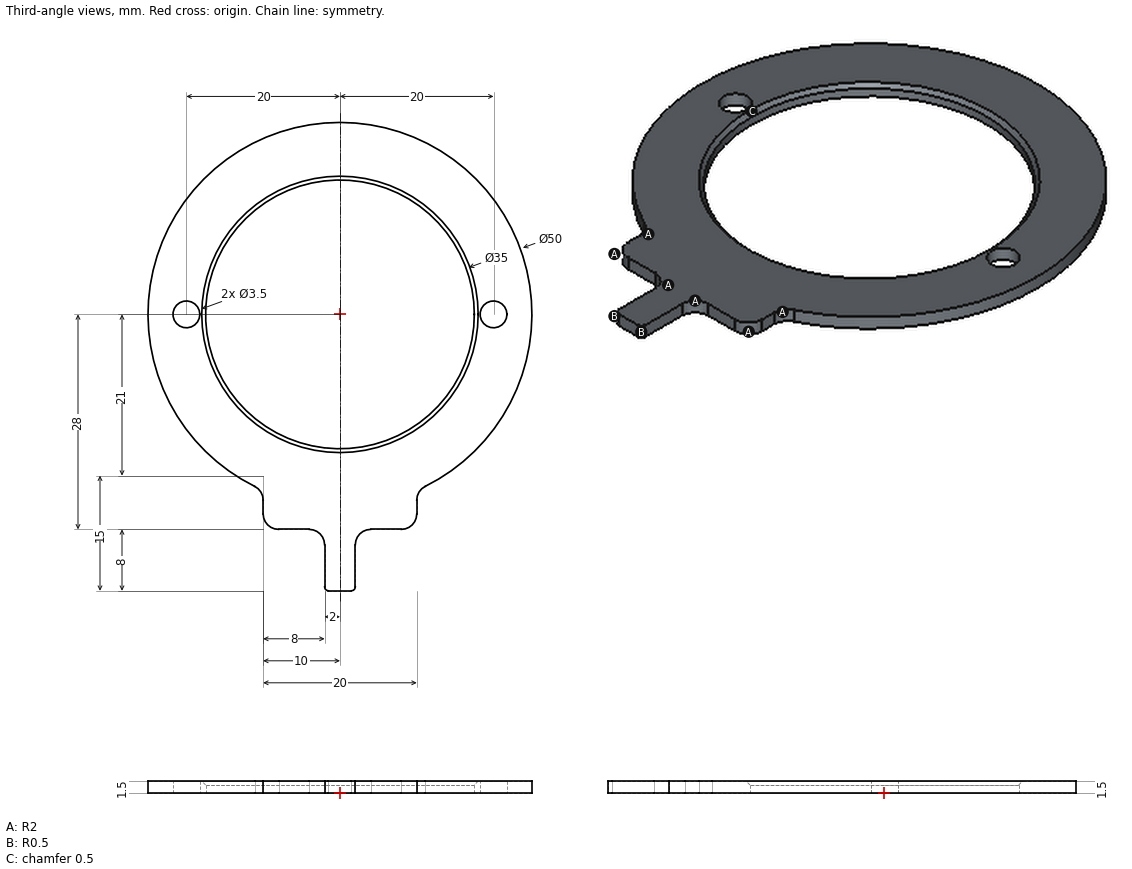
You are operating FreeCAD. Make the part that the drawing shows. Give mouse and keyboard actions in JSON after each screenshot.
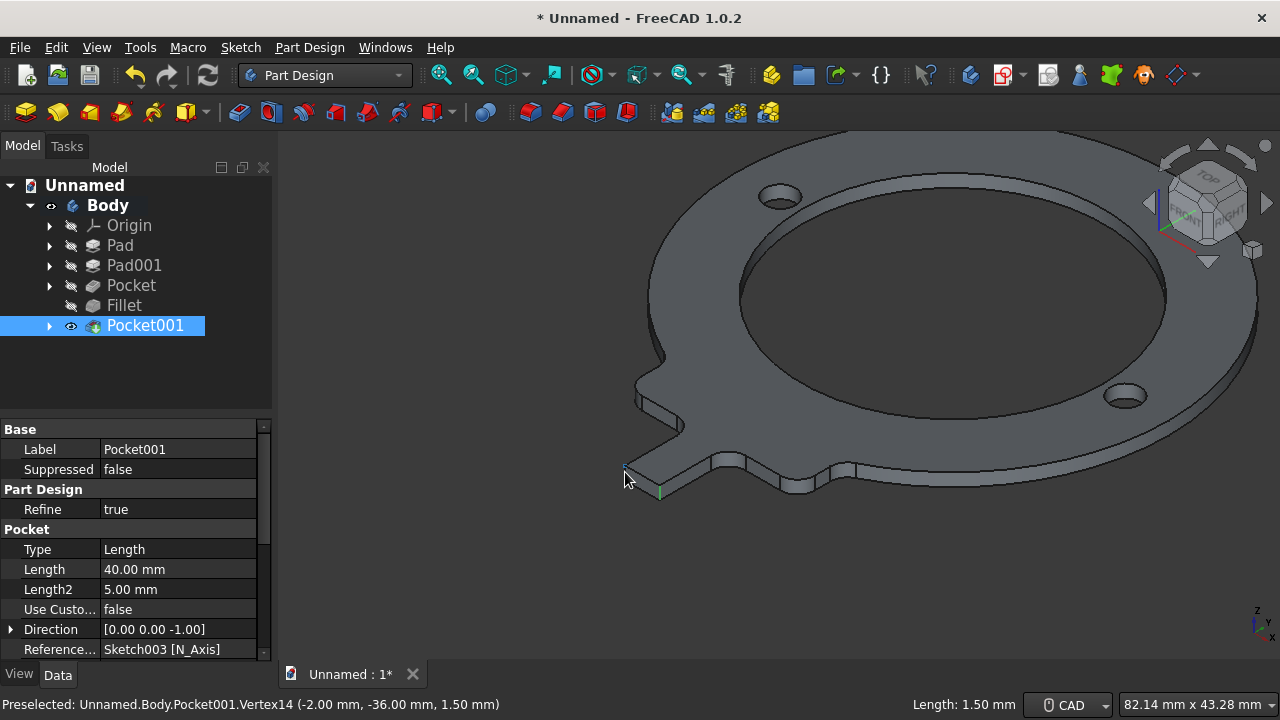
{"action": "left_click", "coordinate": [442, 76]}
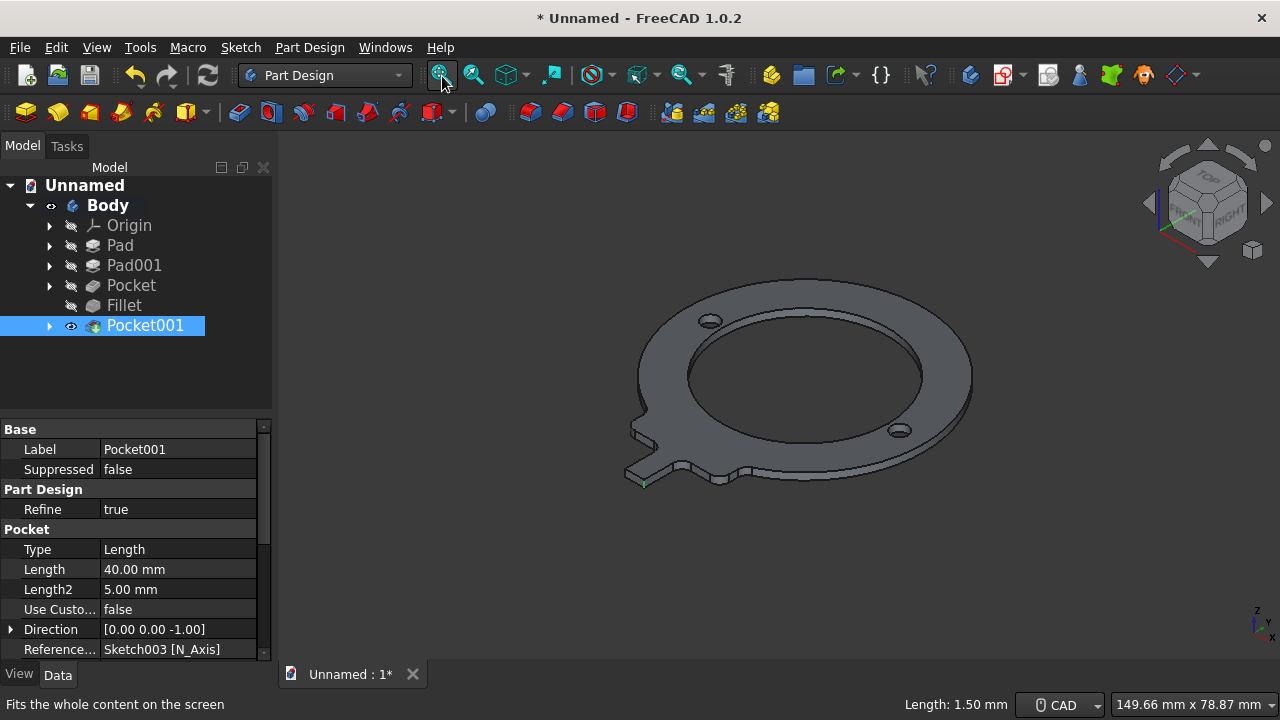
{"action": "key", "text": "1"}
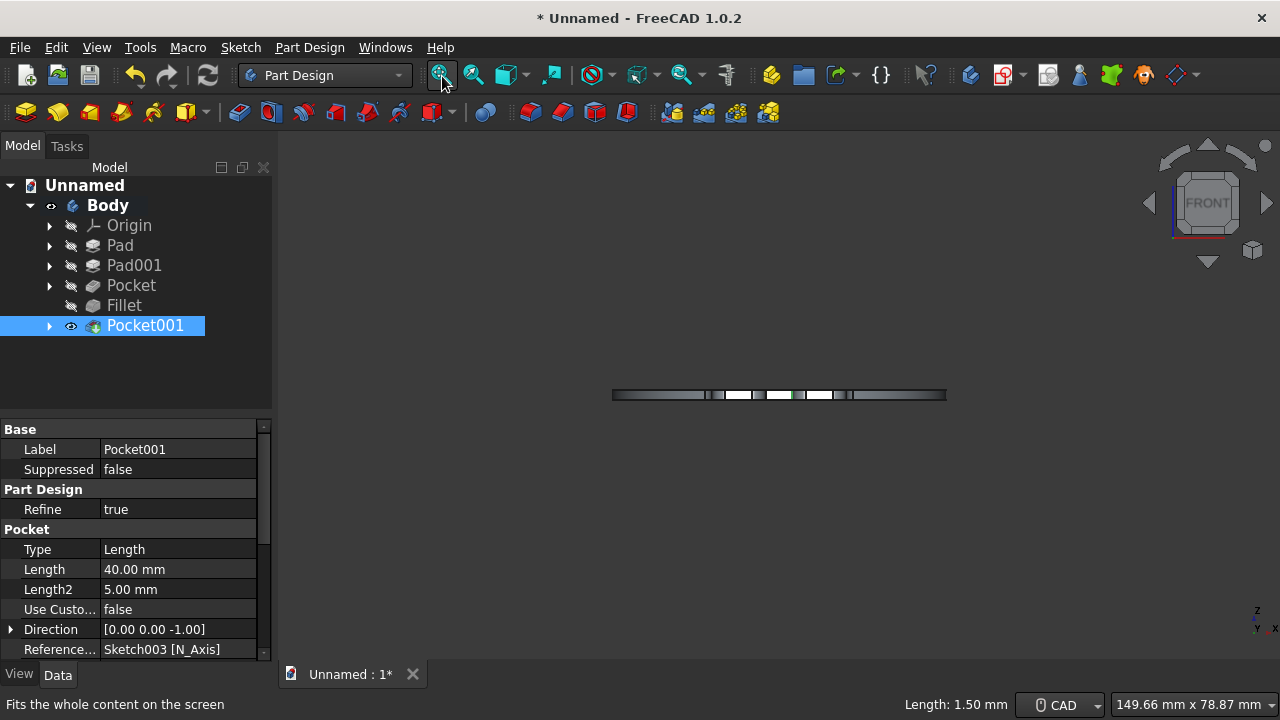
{"action": "left_click", "coordinate": [442, 76]}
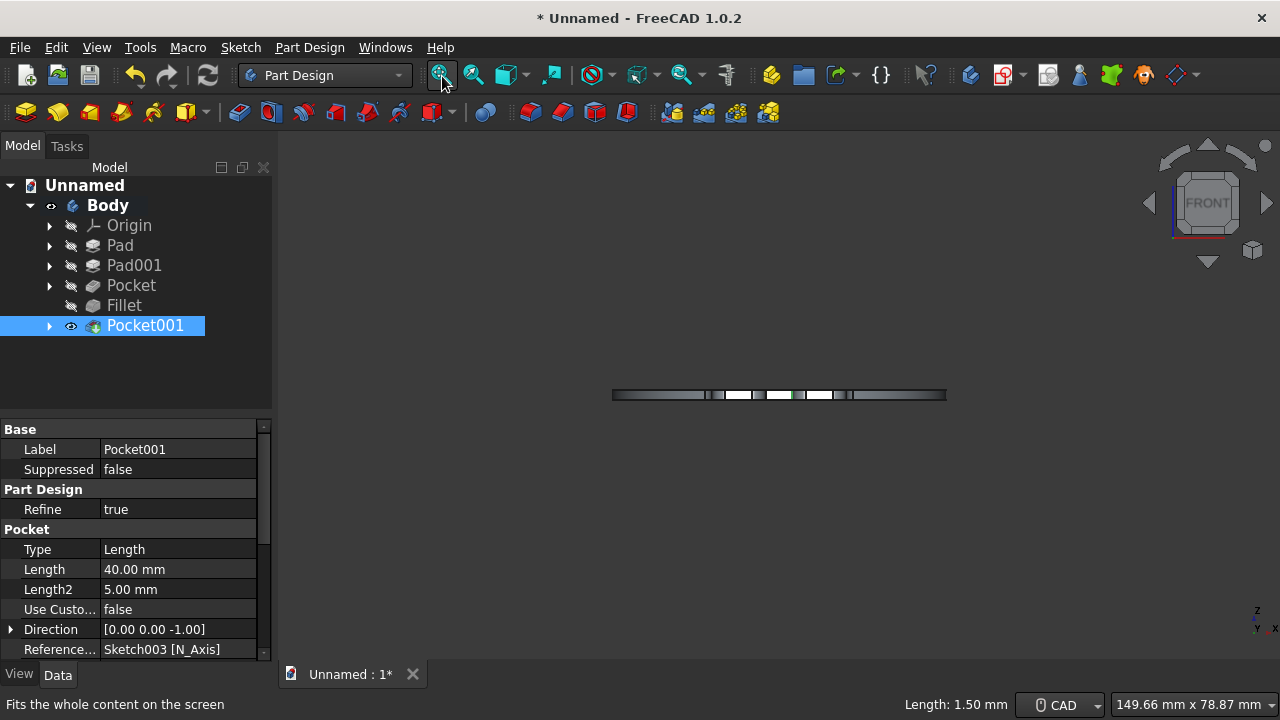
{"action": "scroll", "coordinate": [766, 394], "scroll_direction": "up", "scroll_amount": 7}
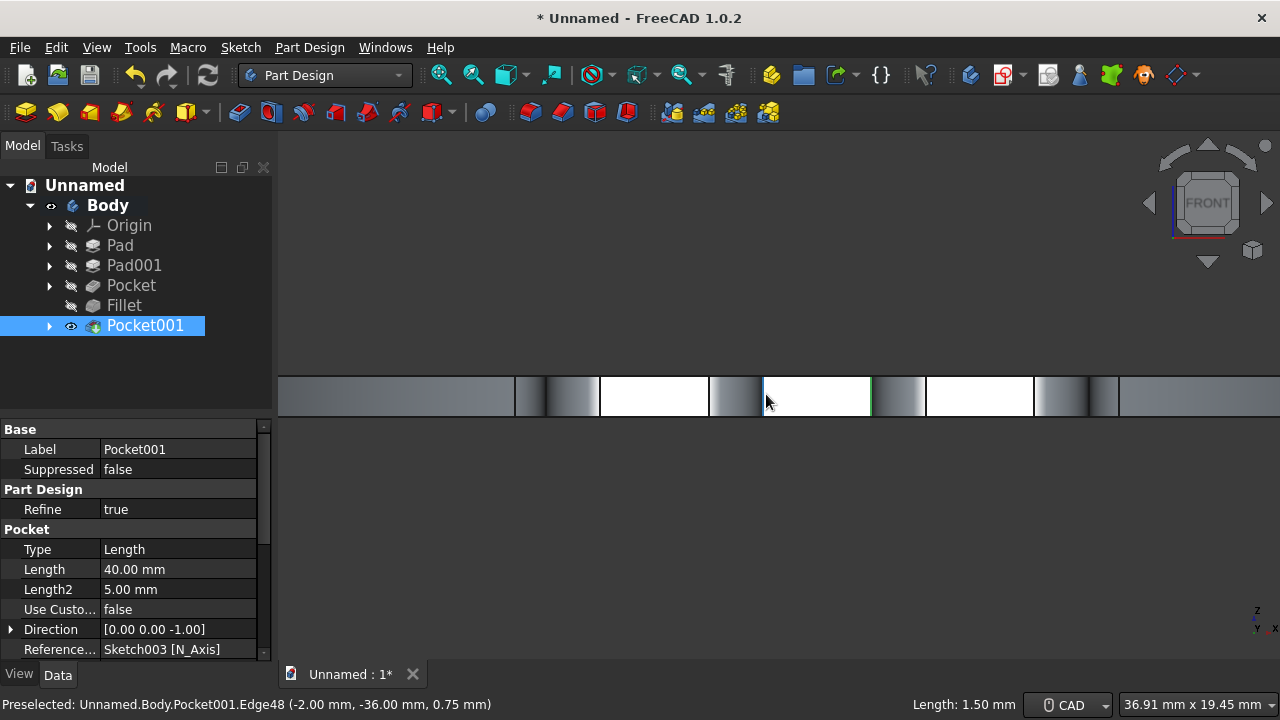
{"action": "left_click", "coordinate": [763, 396], "text": "ctrl"}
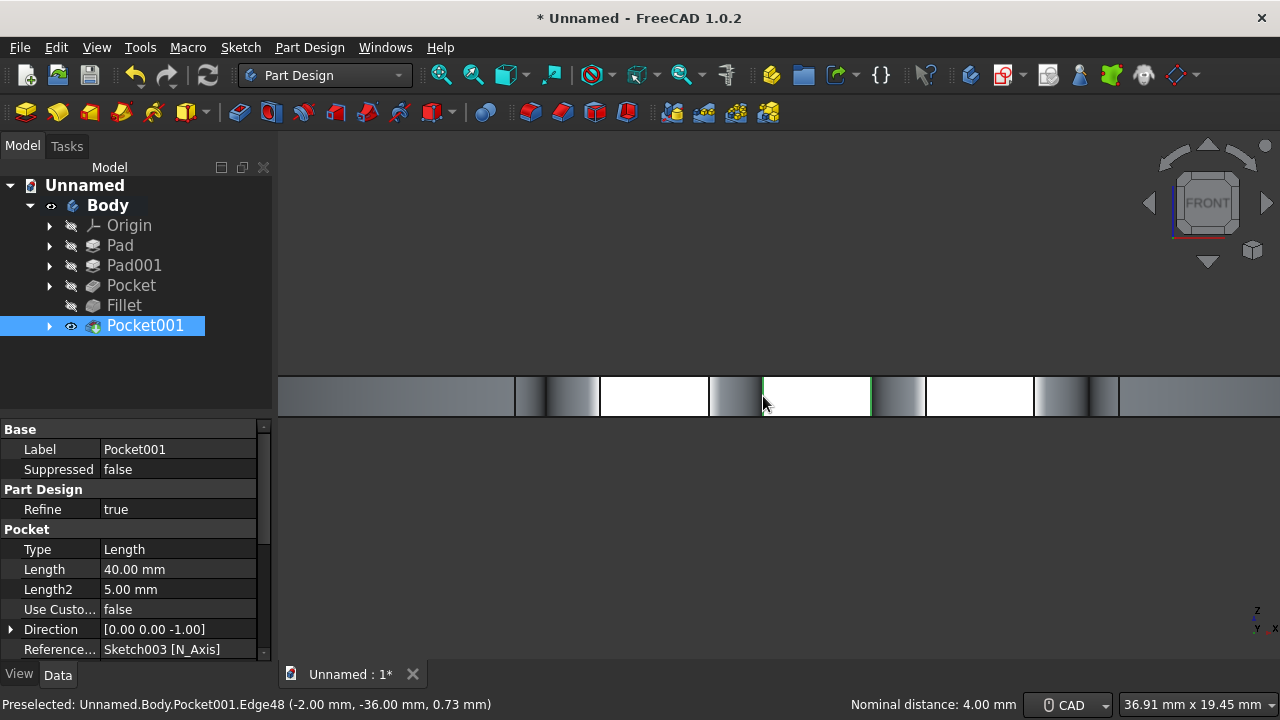
{"action": "left_click", "coordinate": [532, 112]}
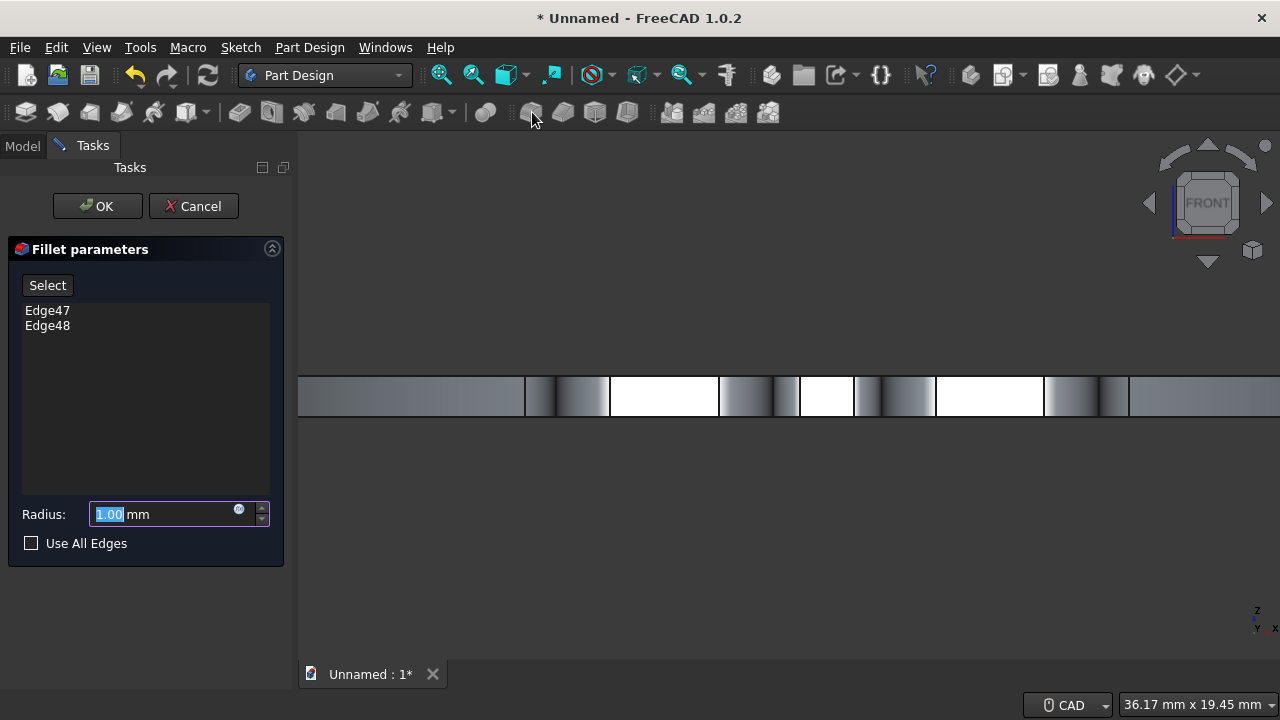
{"action": "type", "text": "0.5"}
{"action": "key", "text": "Tab"}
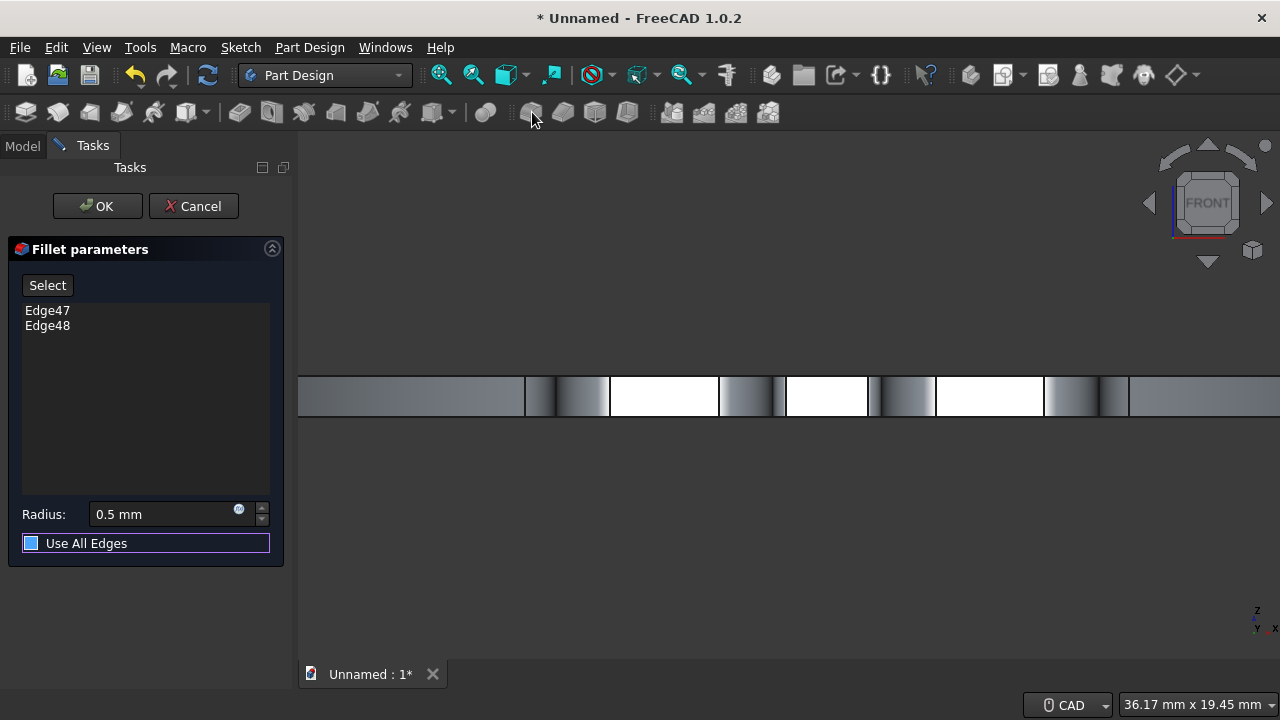
{"action": "left_click", "coordinate": [98, 206]}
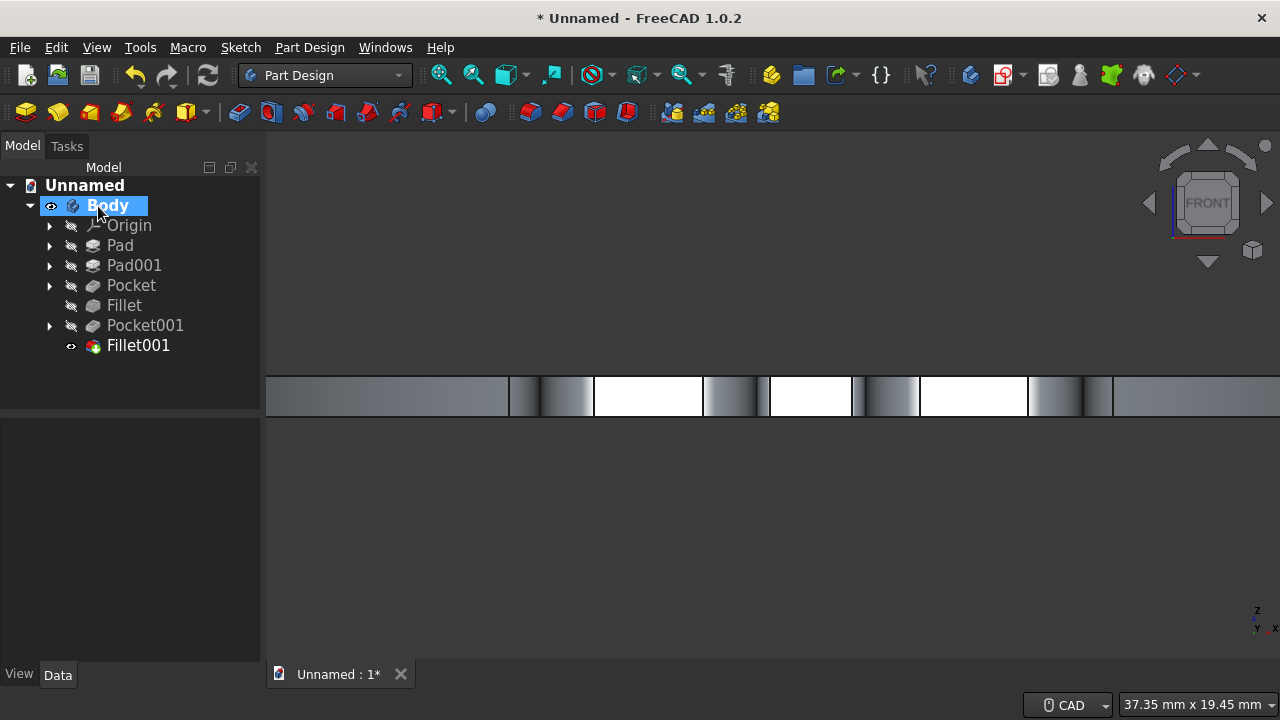
{"action": "left_click", "coordinate": [442, 76]}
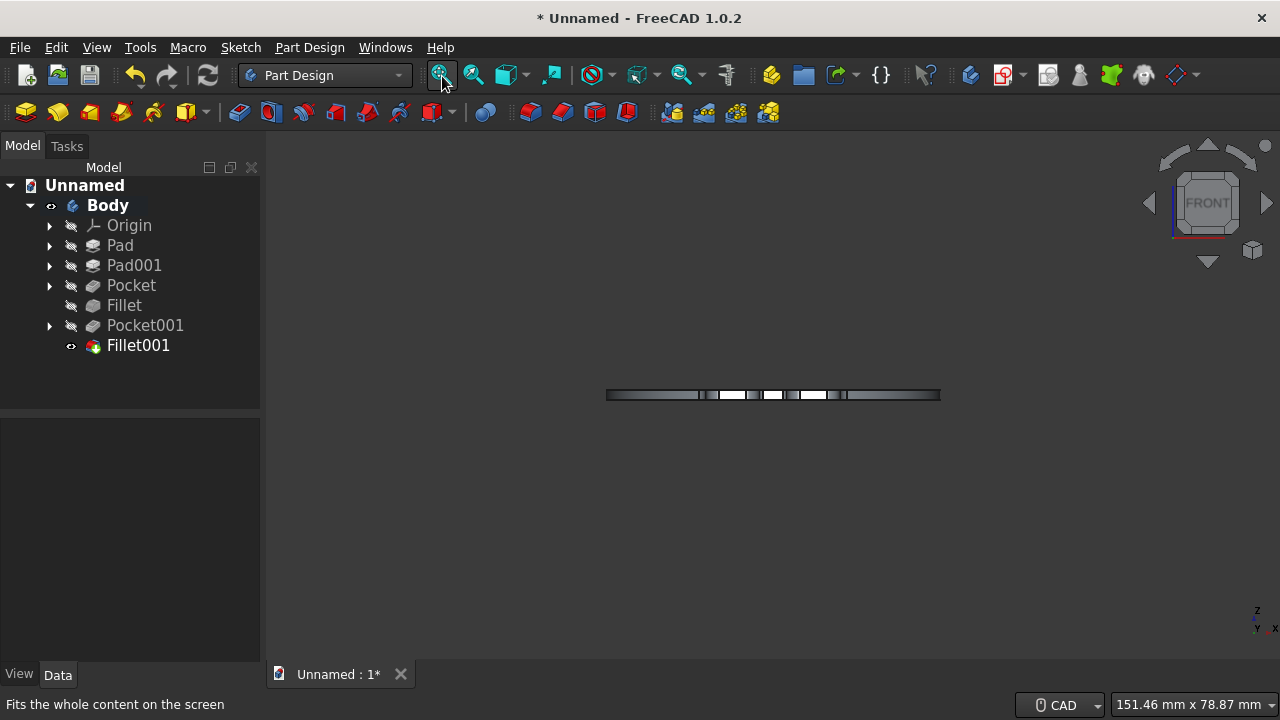
{"action": "key", "text": "0"}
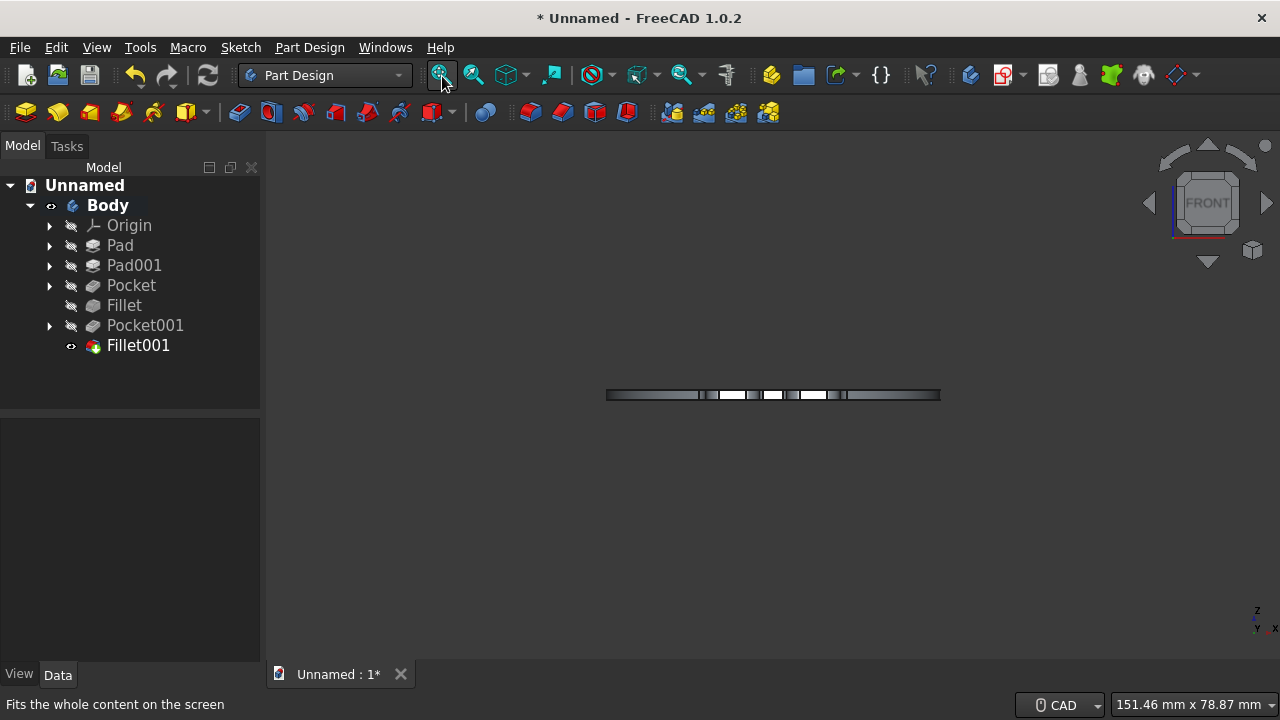
{"action": "left_click", "coordinate": [716, 327]}